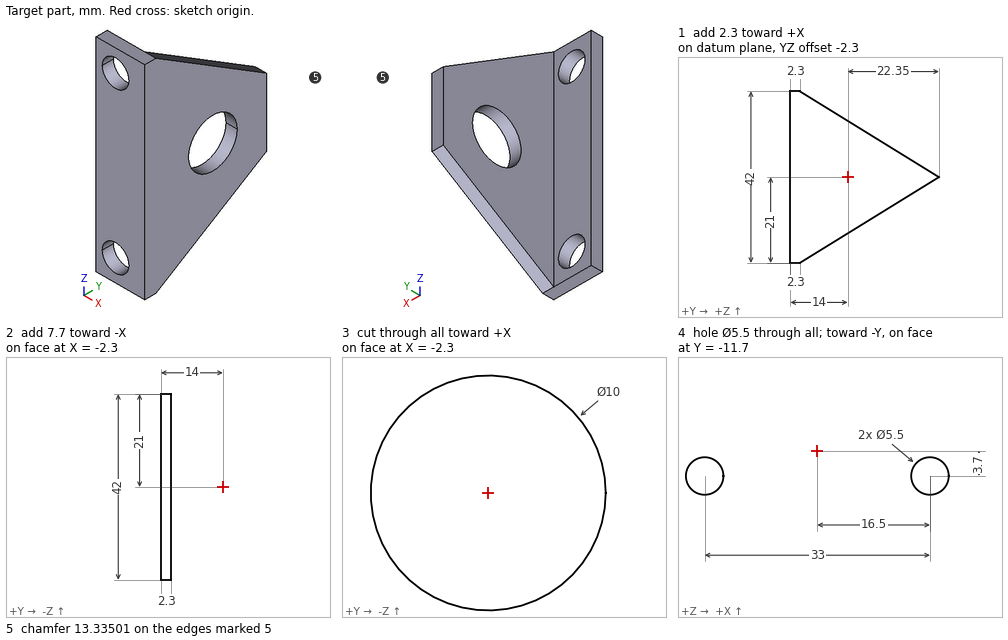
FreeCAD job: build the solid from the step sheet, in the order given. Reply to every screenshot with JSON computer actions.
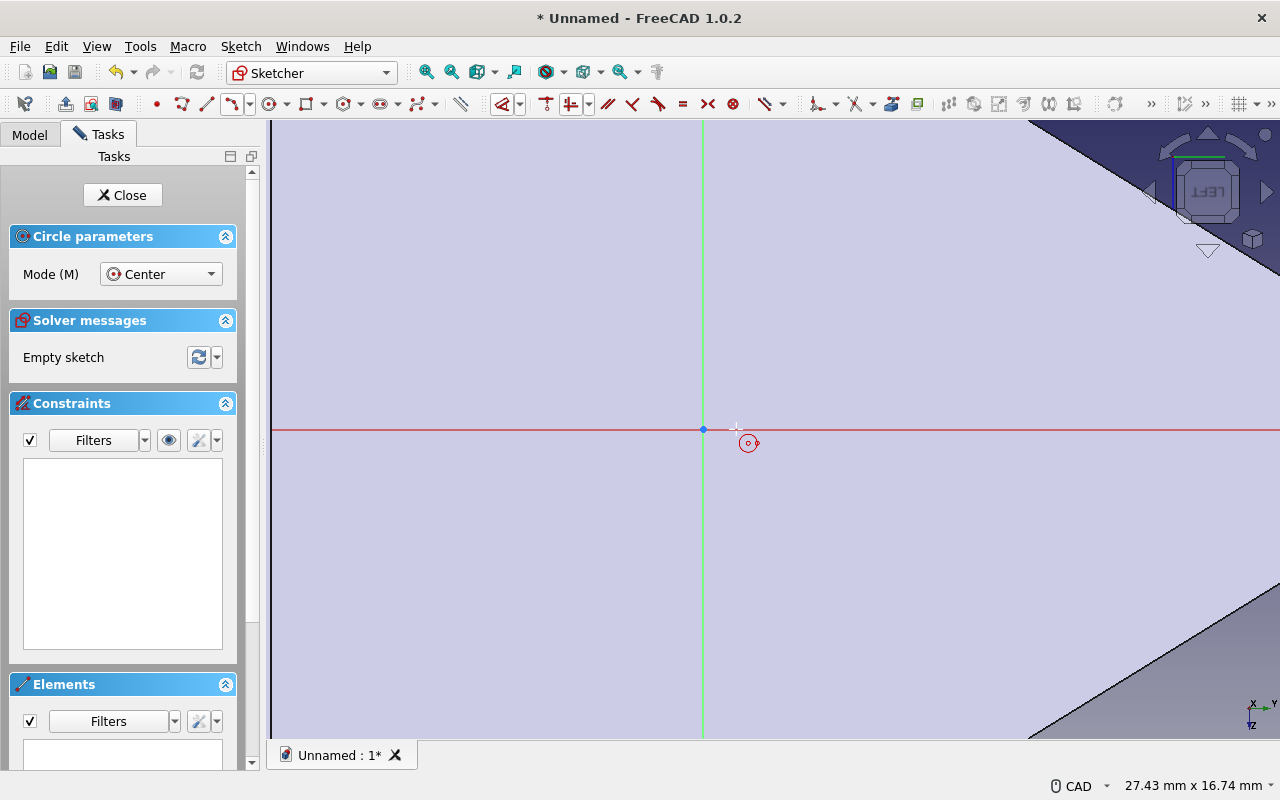
{"action": "left_click", "coordinate": [703, 429]}
{"action": "left_click", "coordinate": [834, 299]}
{"action": "key", "text": "Escape"}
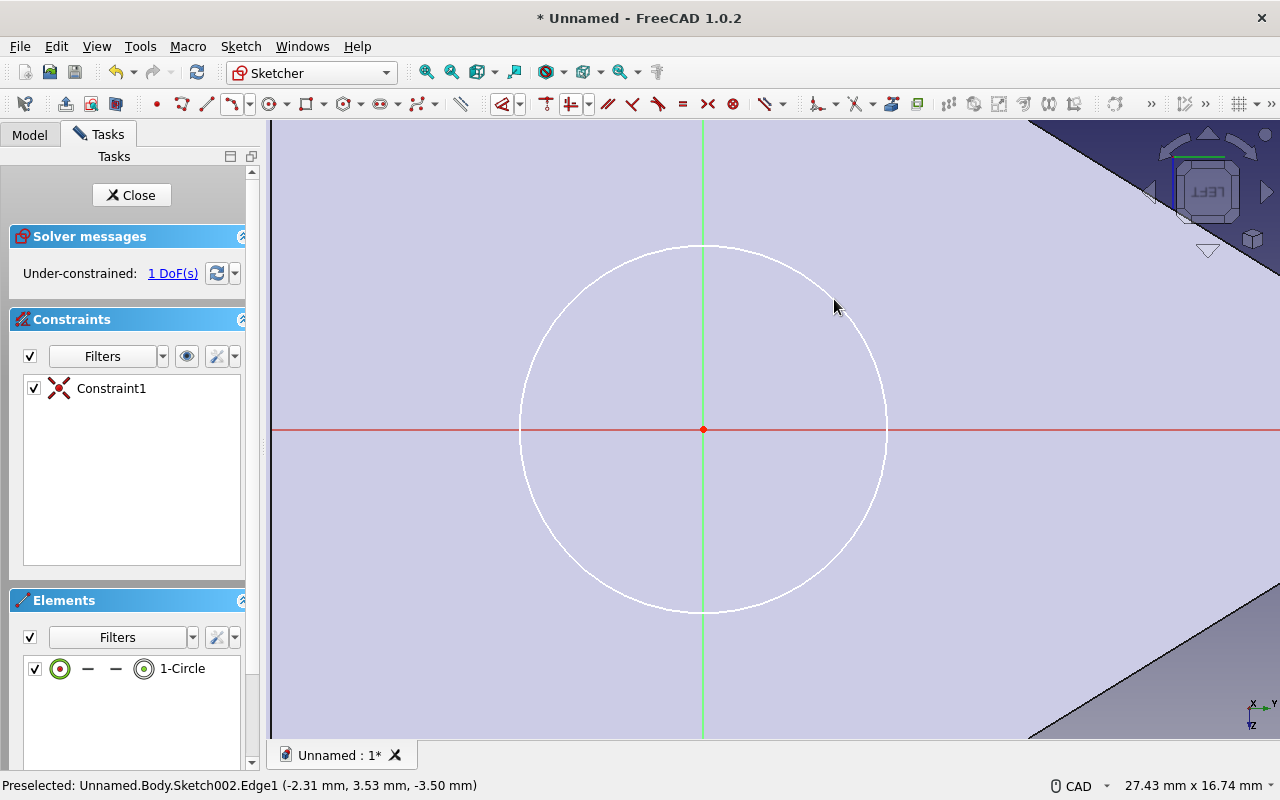
{"action": "left_click", "coordinate": [833, 299]}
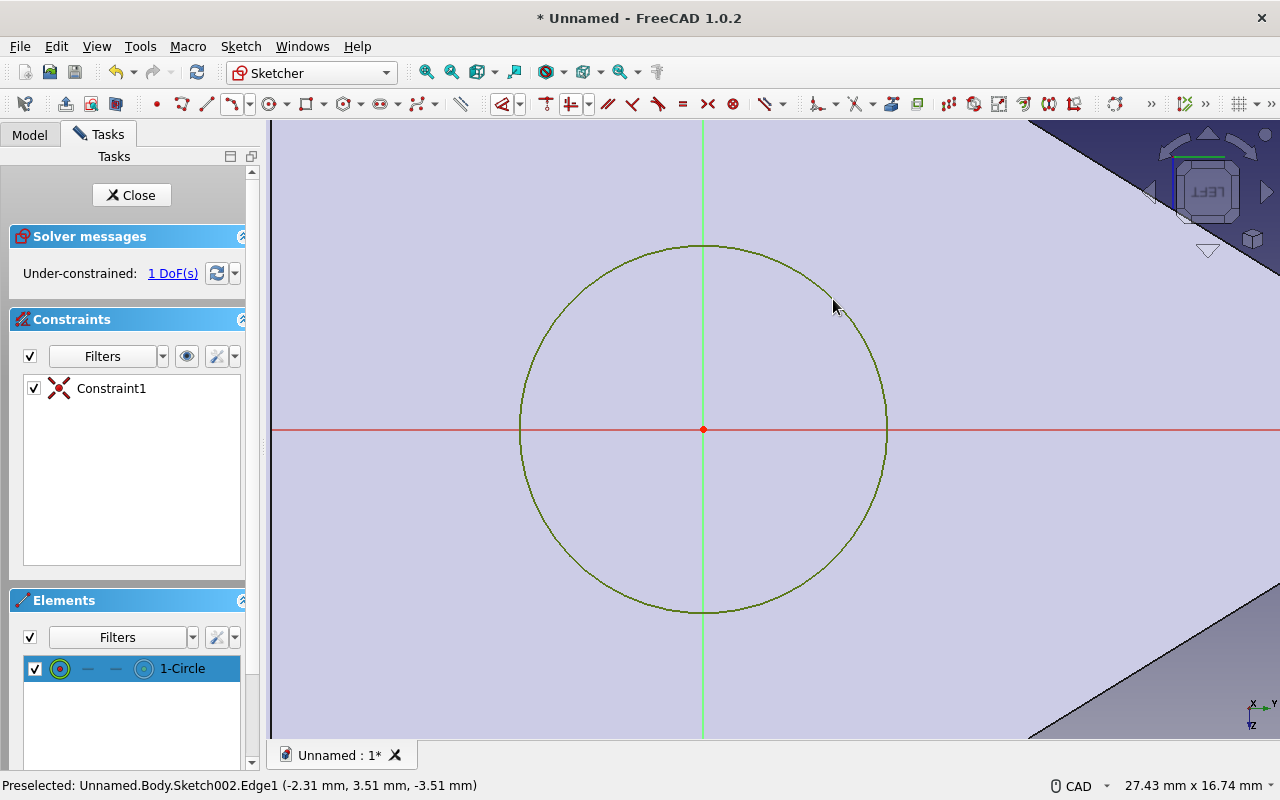
{"action": "key", "text": "k o"}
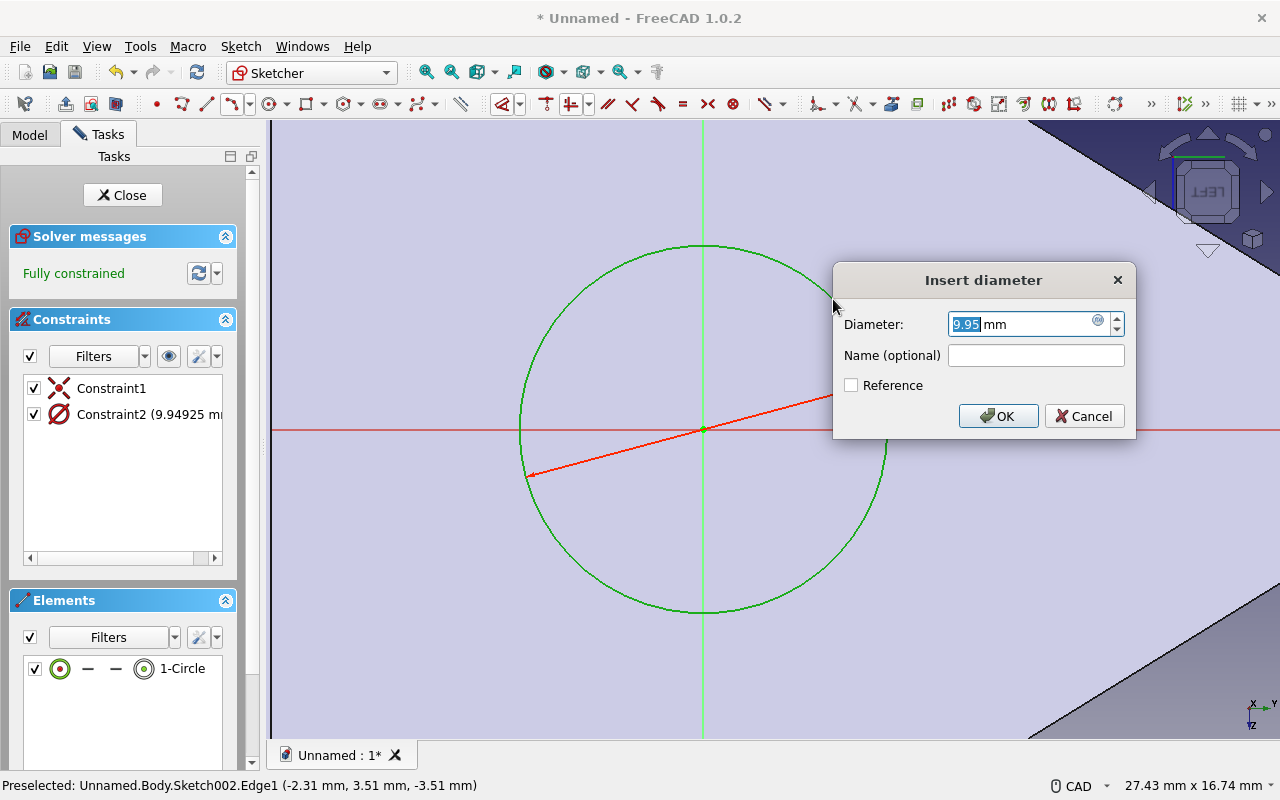
{"action": "type", "text": "10"}
{"action": "key", "text": "Return"}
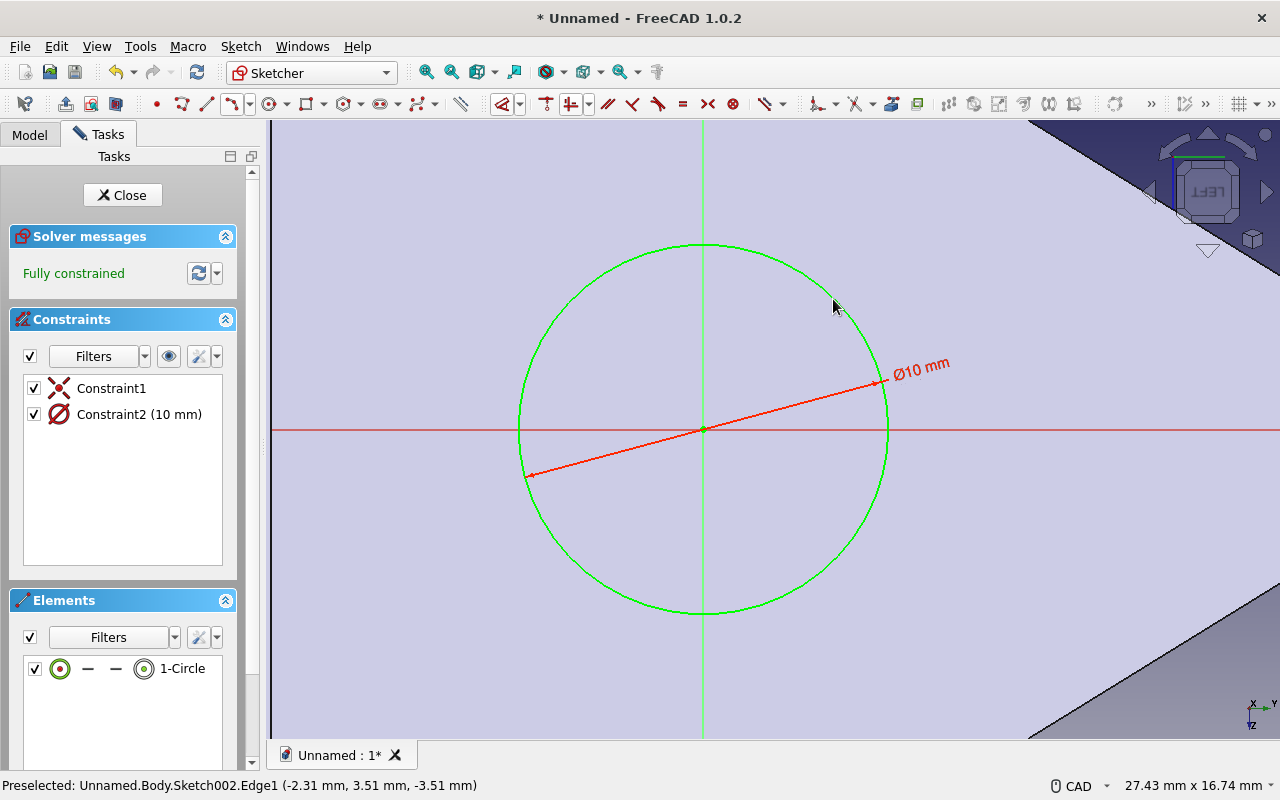
{"action": "left_click", "coordinate": [123, 195]}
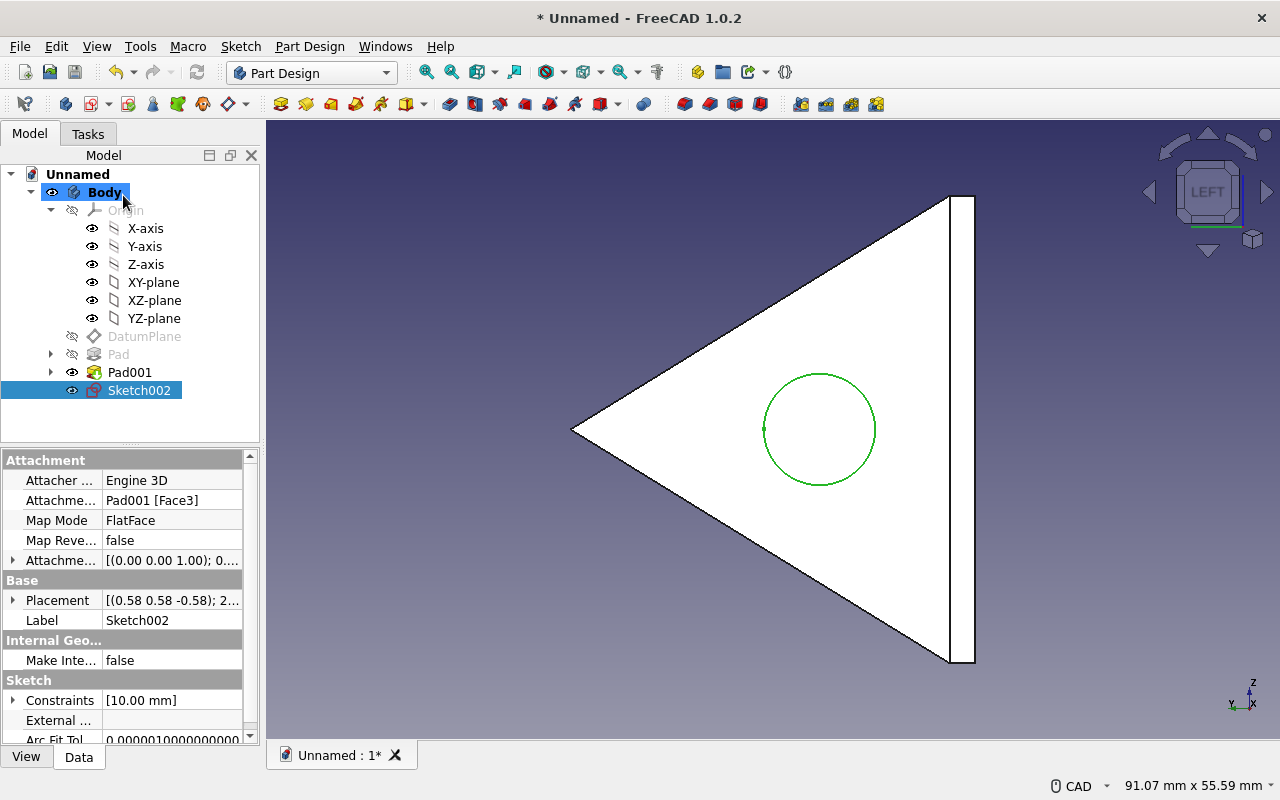
{"action": "left_click", "coordinate": [450, 104]}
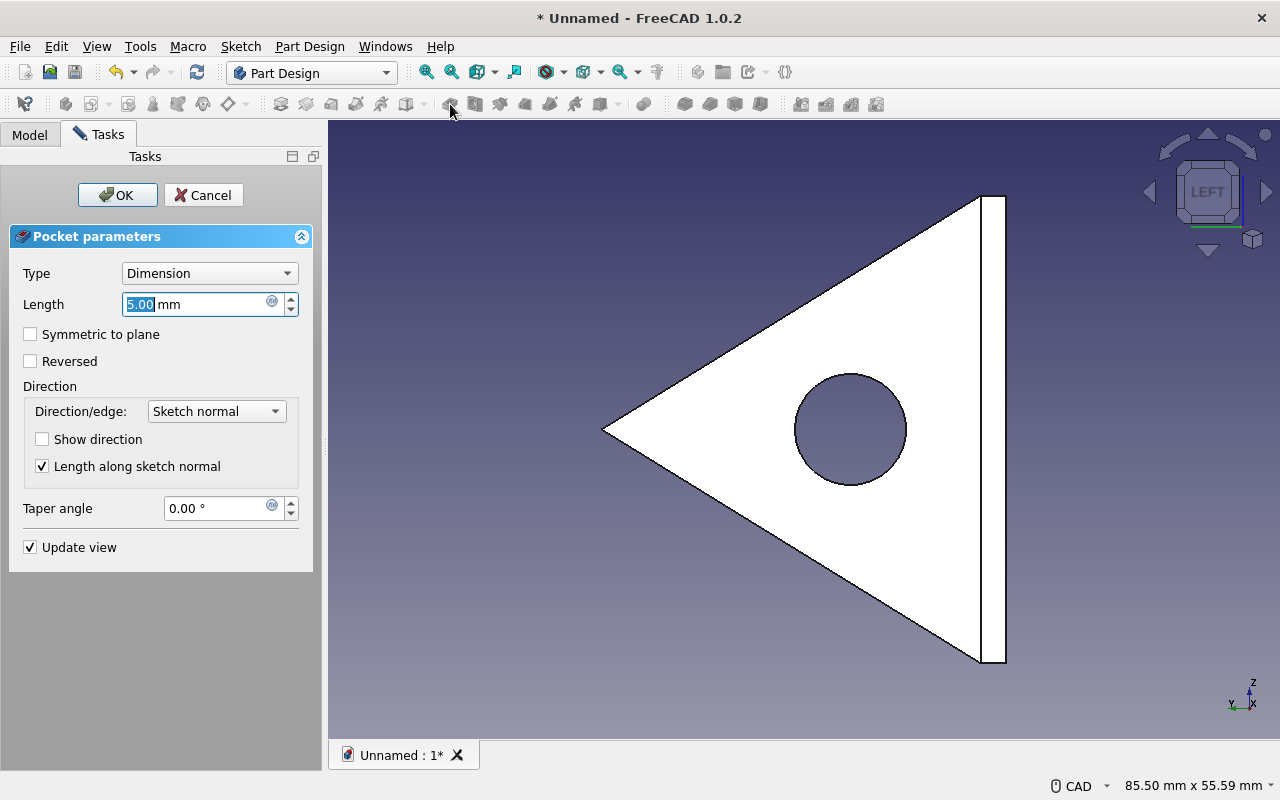
{"action": "left_click", "coordinate": [210, 274]}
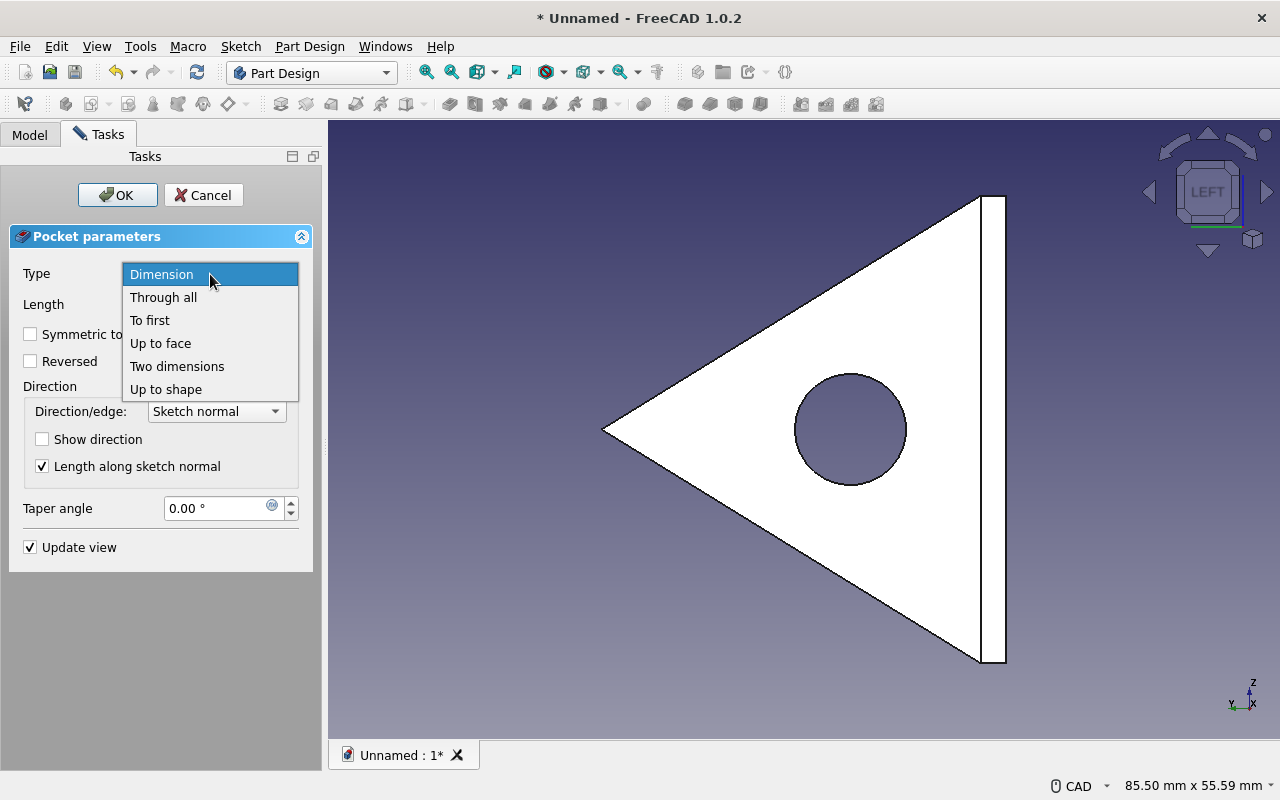
{"action": "left_click", "coordinate": [208, 298]}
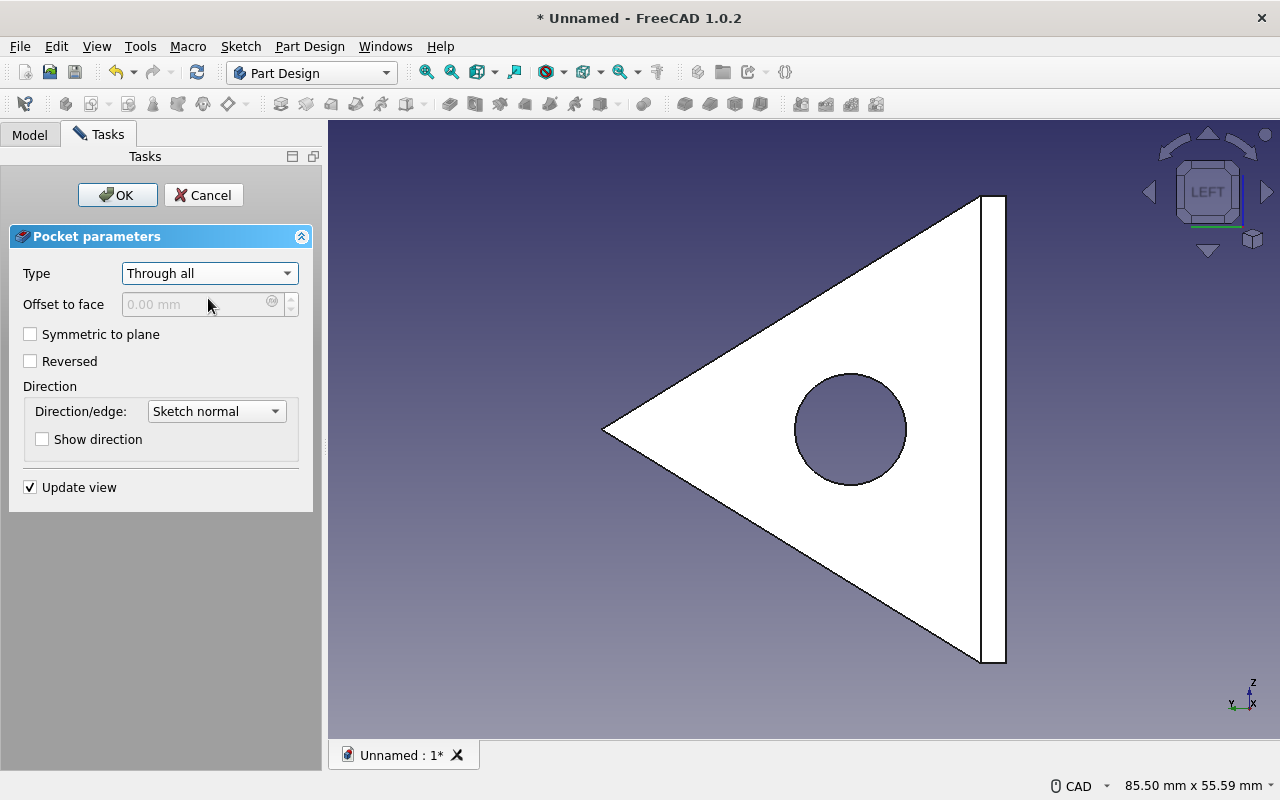
{"action": "left_click", "coordinate": [118, 195]}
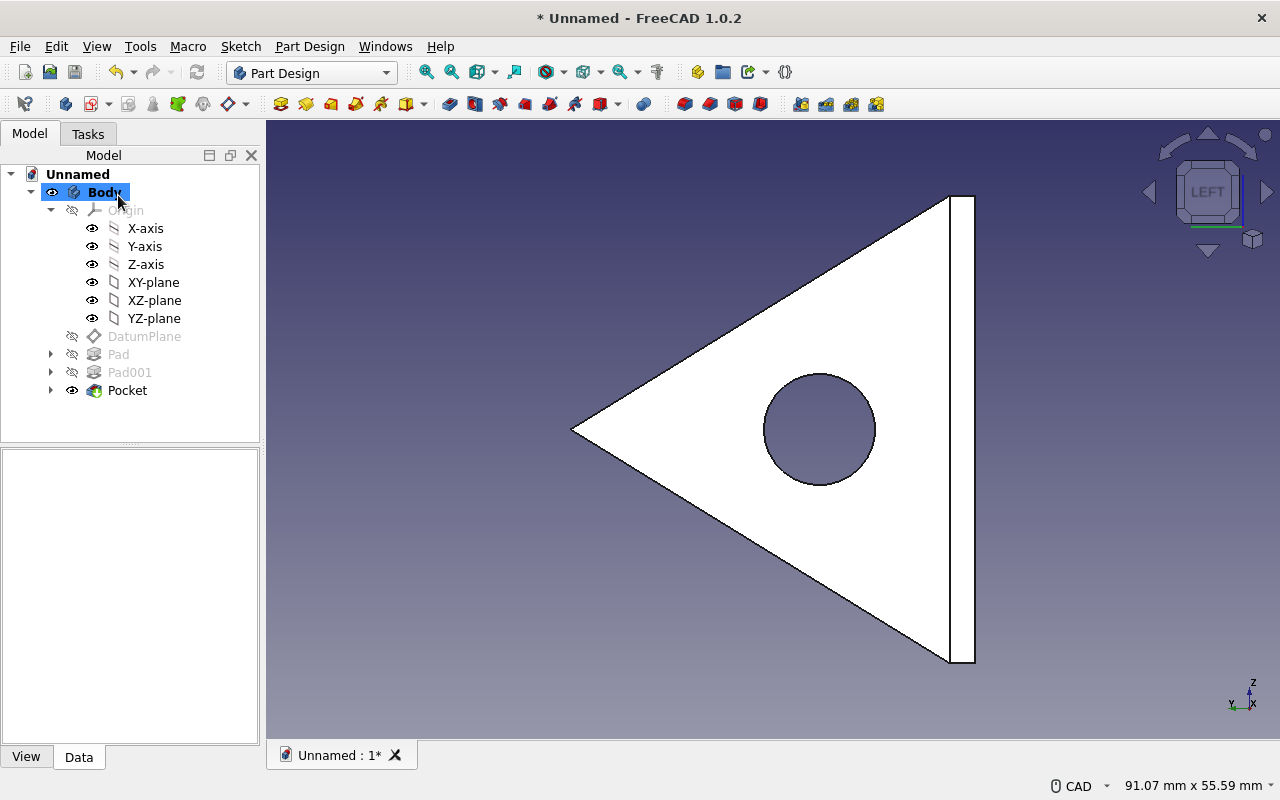
{"action": "key", "text": "4"}